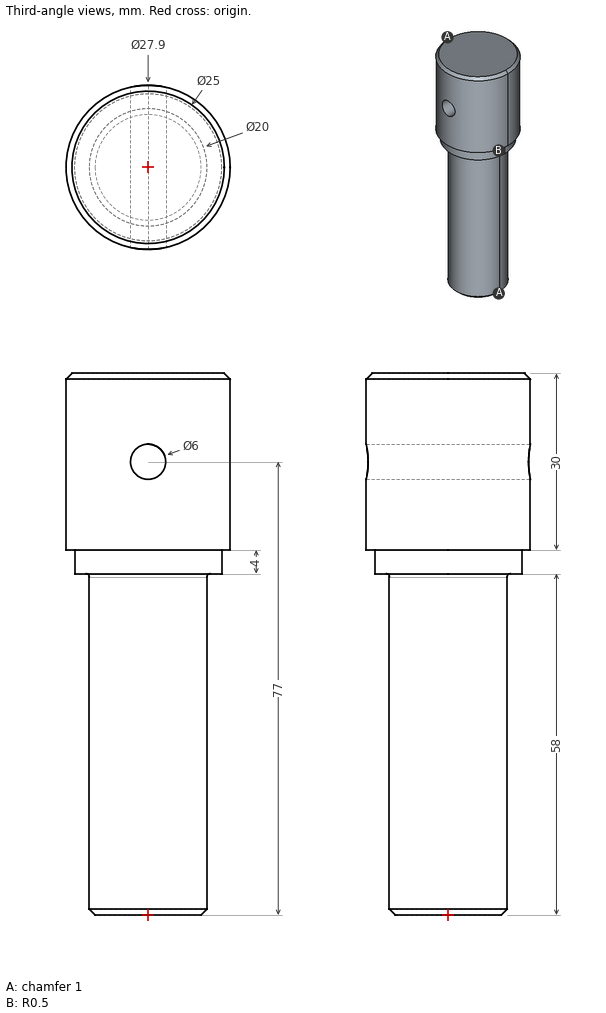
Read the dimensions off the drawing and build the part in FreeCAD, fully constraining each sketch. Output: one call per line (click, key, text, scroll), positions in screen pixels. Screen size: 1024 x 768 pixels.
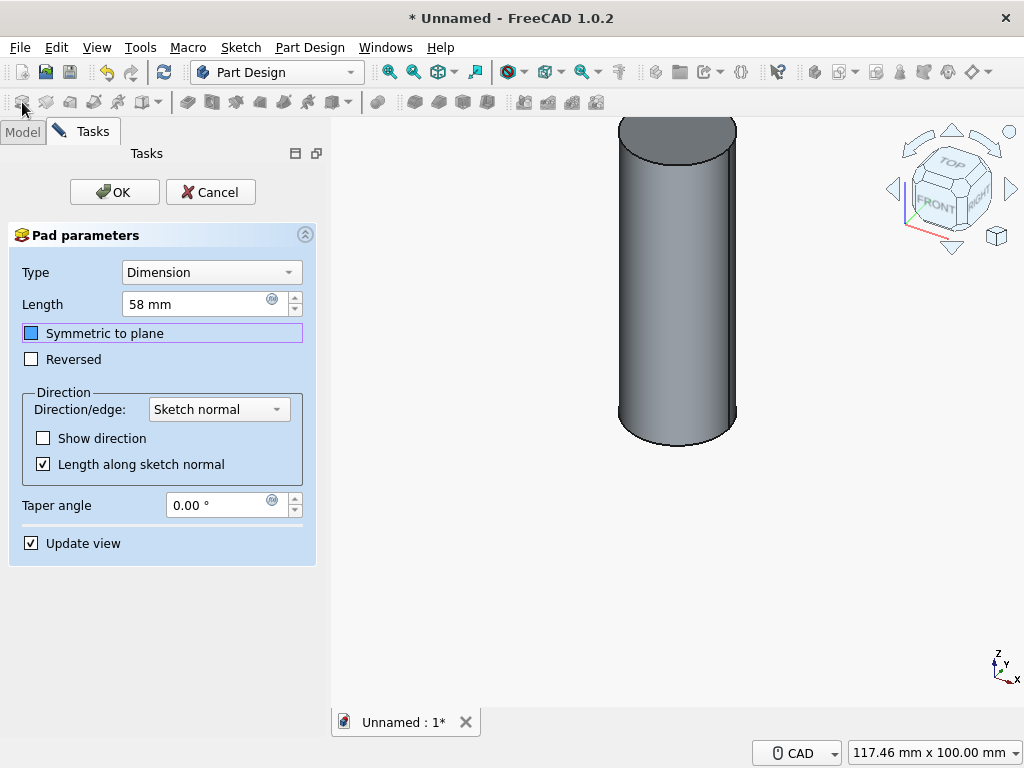
click(115, 192)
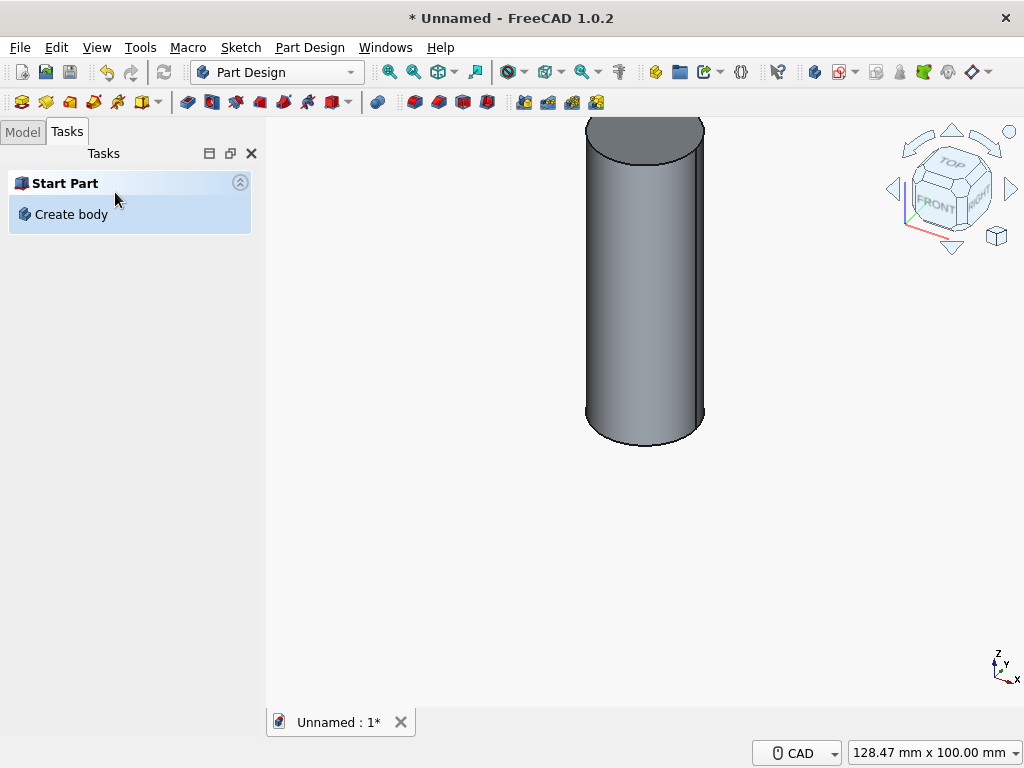
click(390, 72)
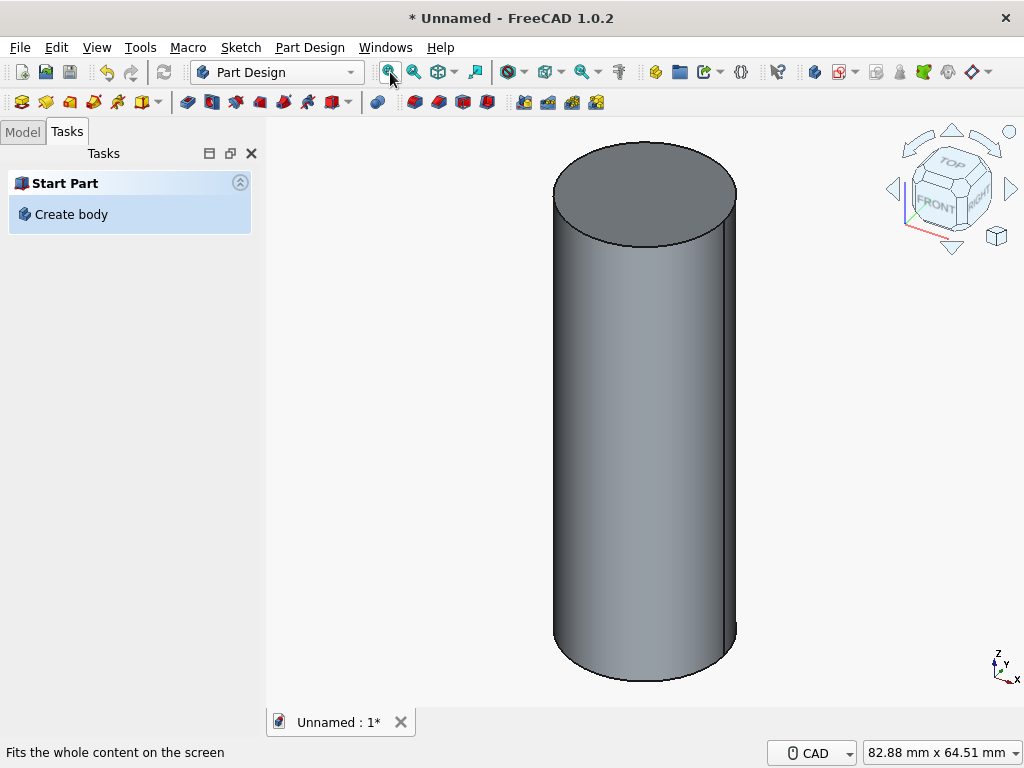
click(645, 194)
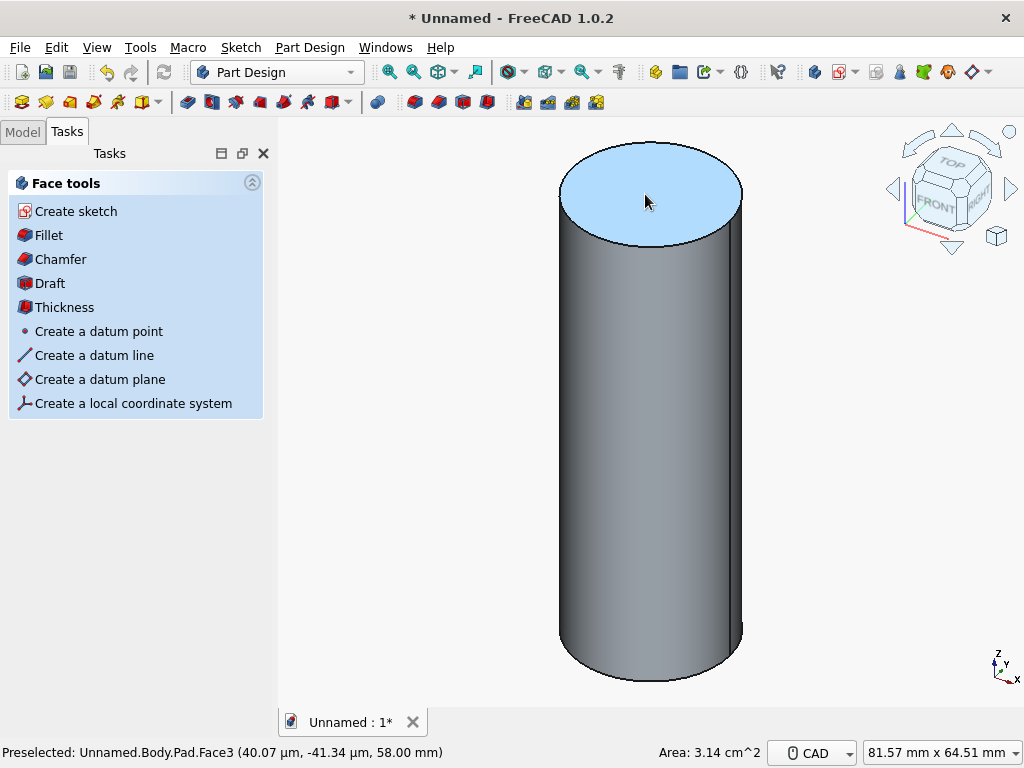
click(840, 72)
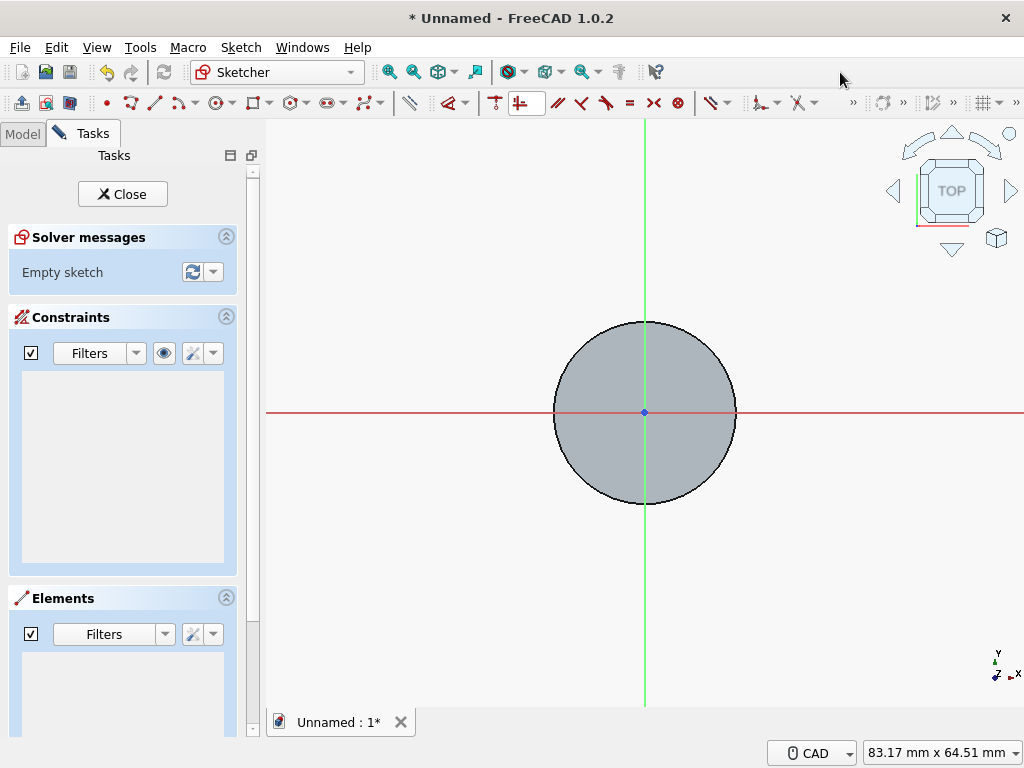
scroll(784, 413, up, 2)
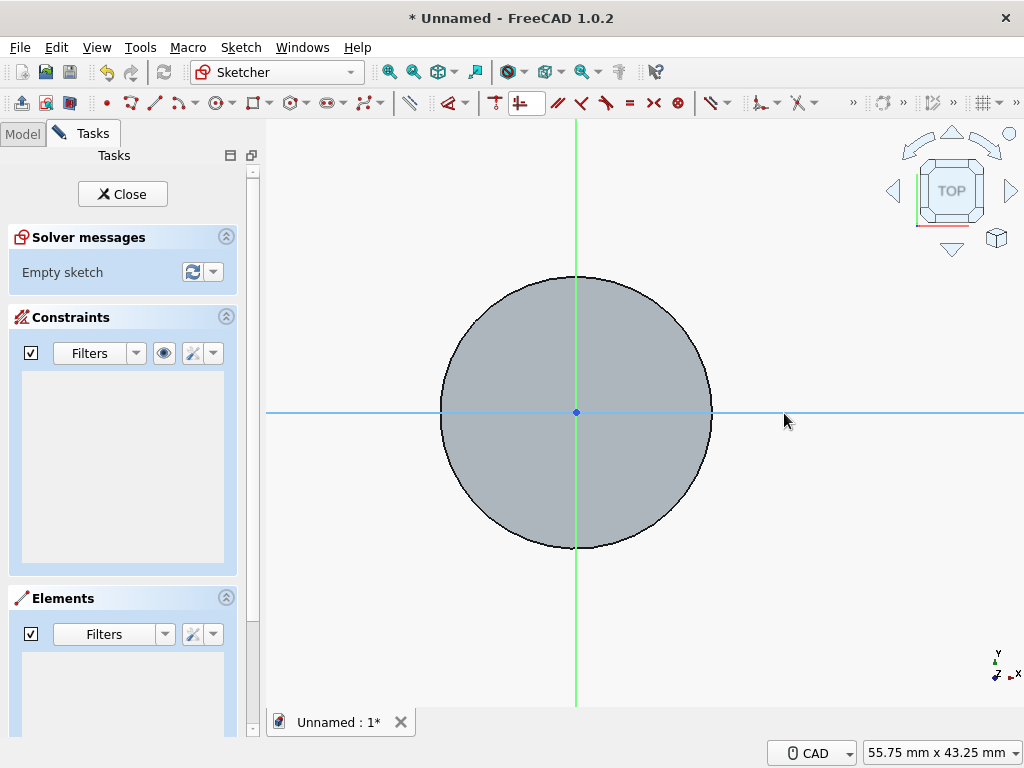
click(216, 104)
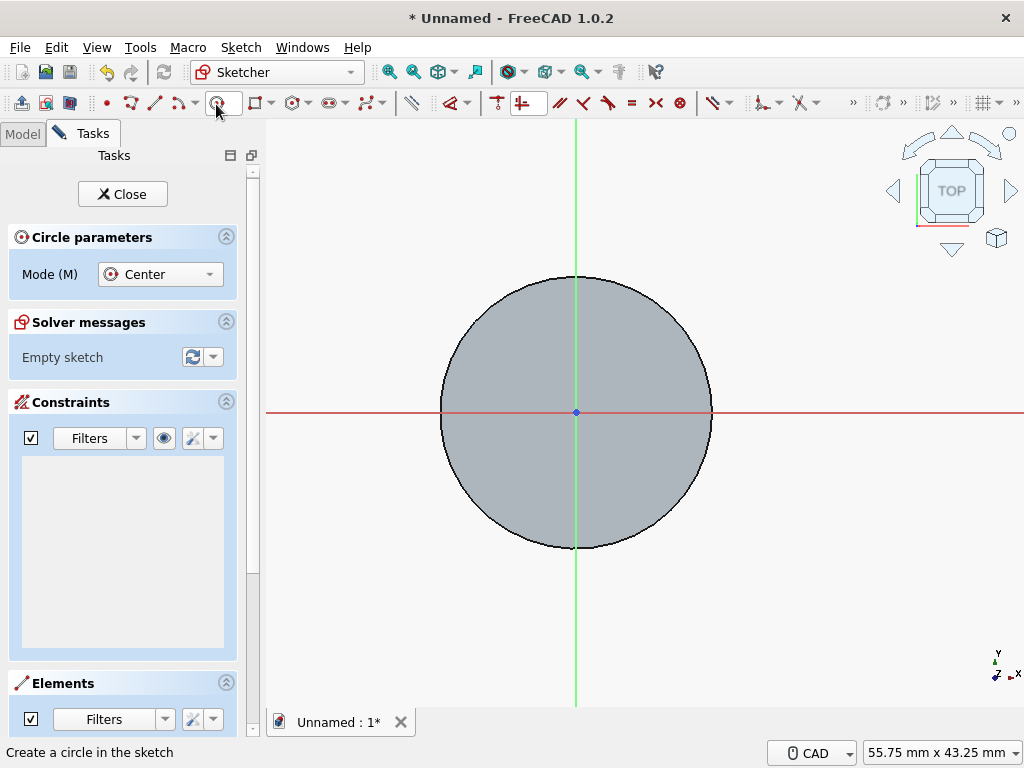
click(576, 413)
click(696, 293)
key(Escape)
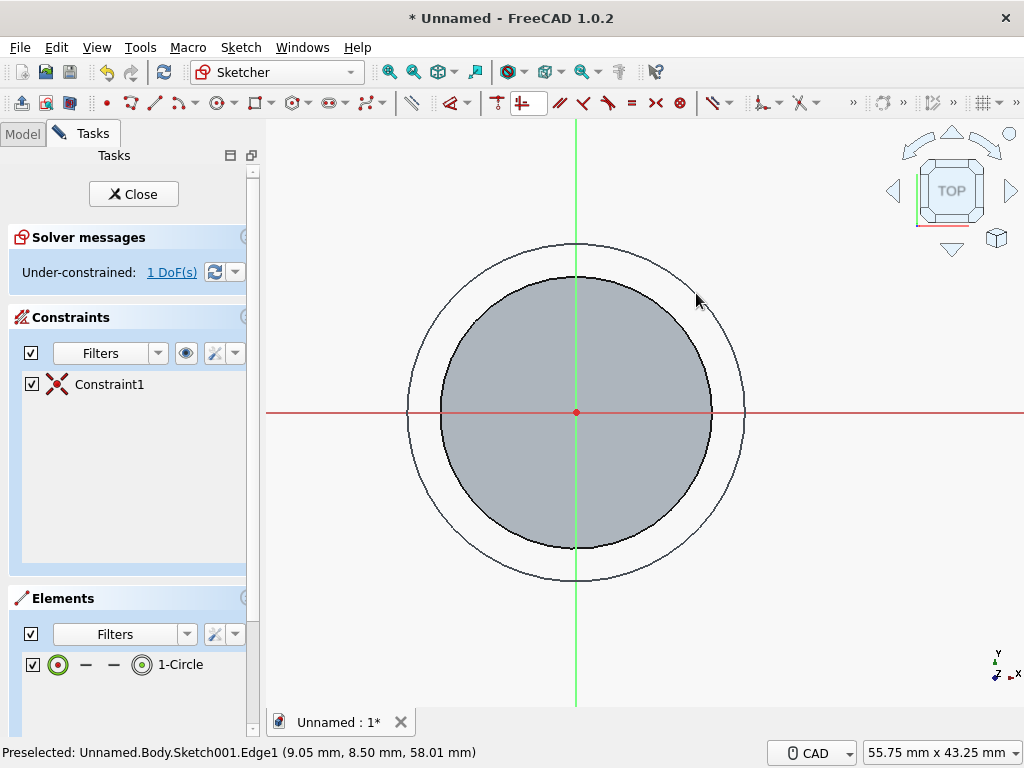
click(450, 104)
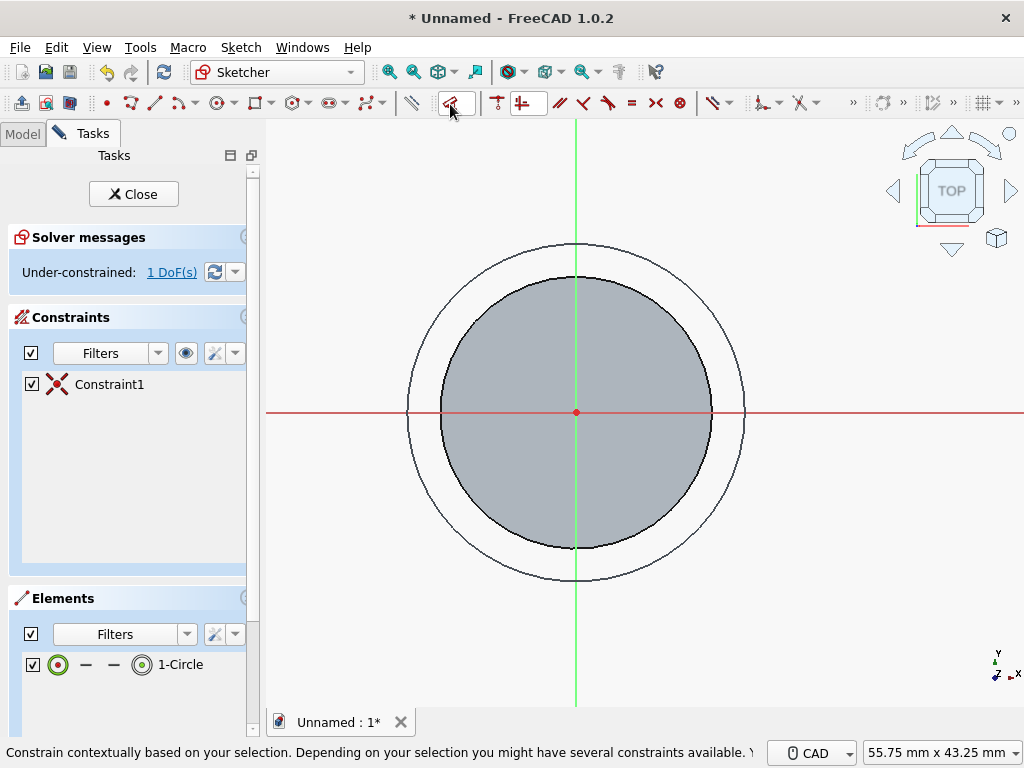
click(695, 293)
click(718, 270)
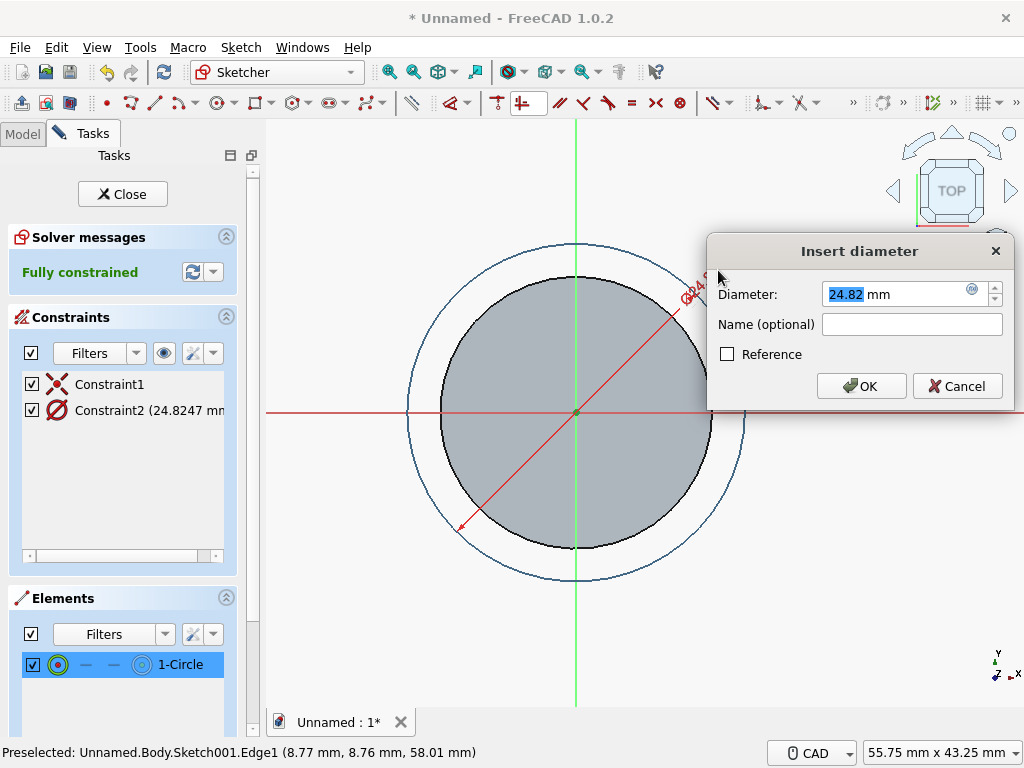
text(25)
key(Return)
key(Escape)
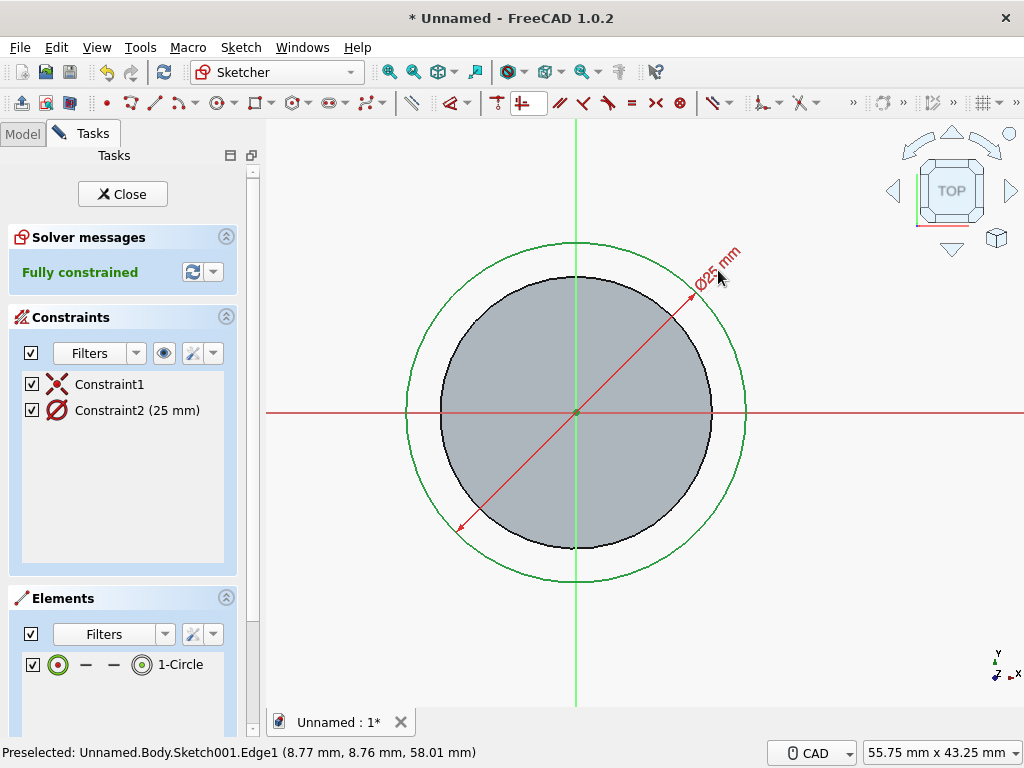
click(123, 194)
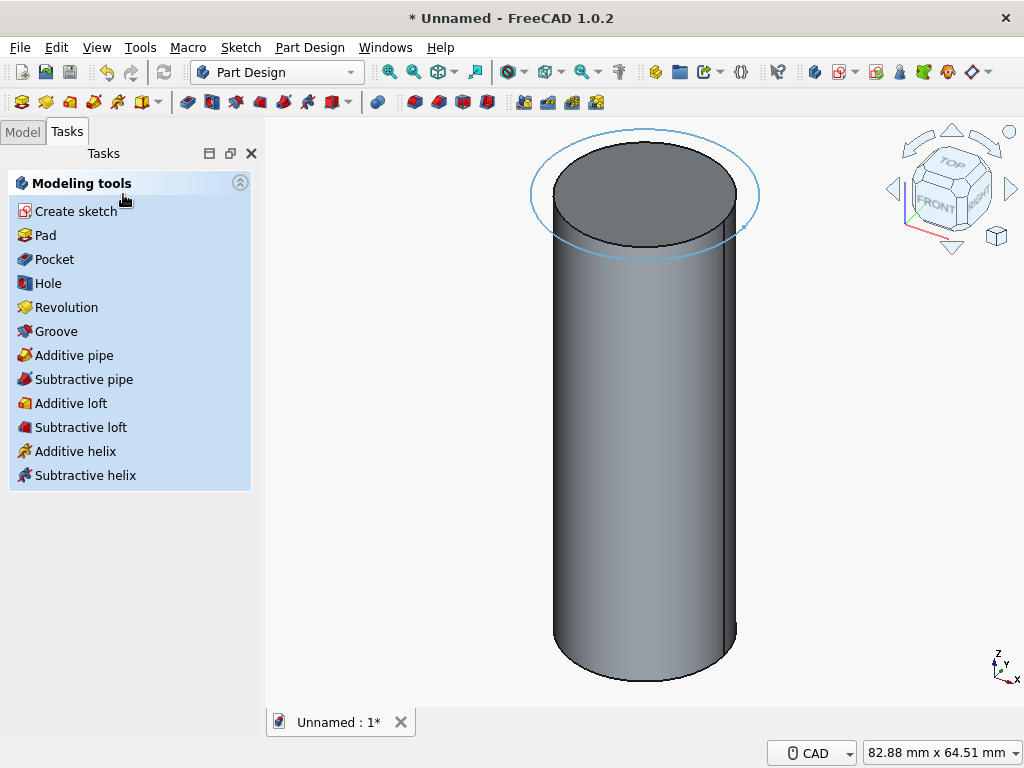
click(22, 102)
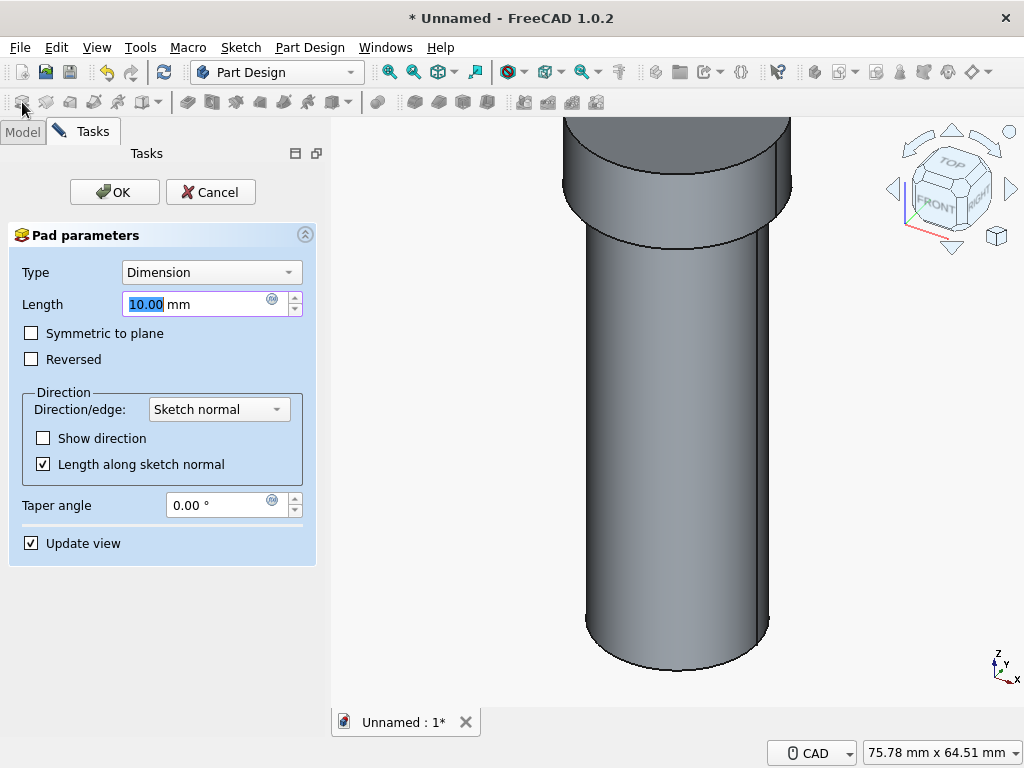
text(4)
key(Tab)